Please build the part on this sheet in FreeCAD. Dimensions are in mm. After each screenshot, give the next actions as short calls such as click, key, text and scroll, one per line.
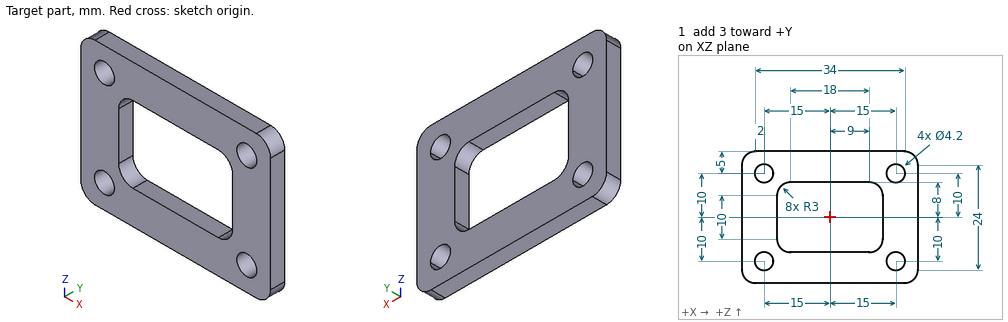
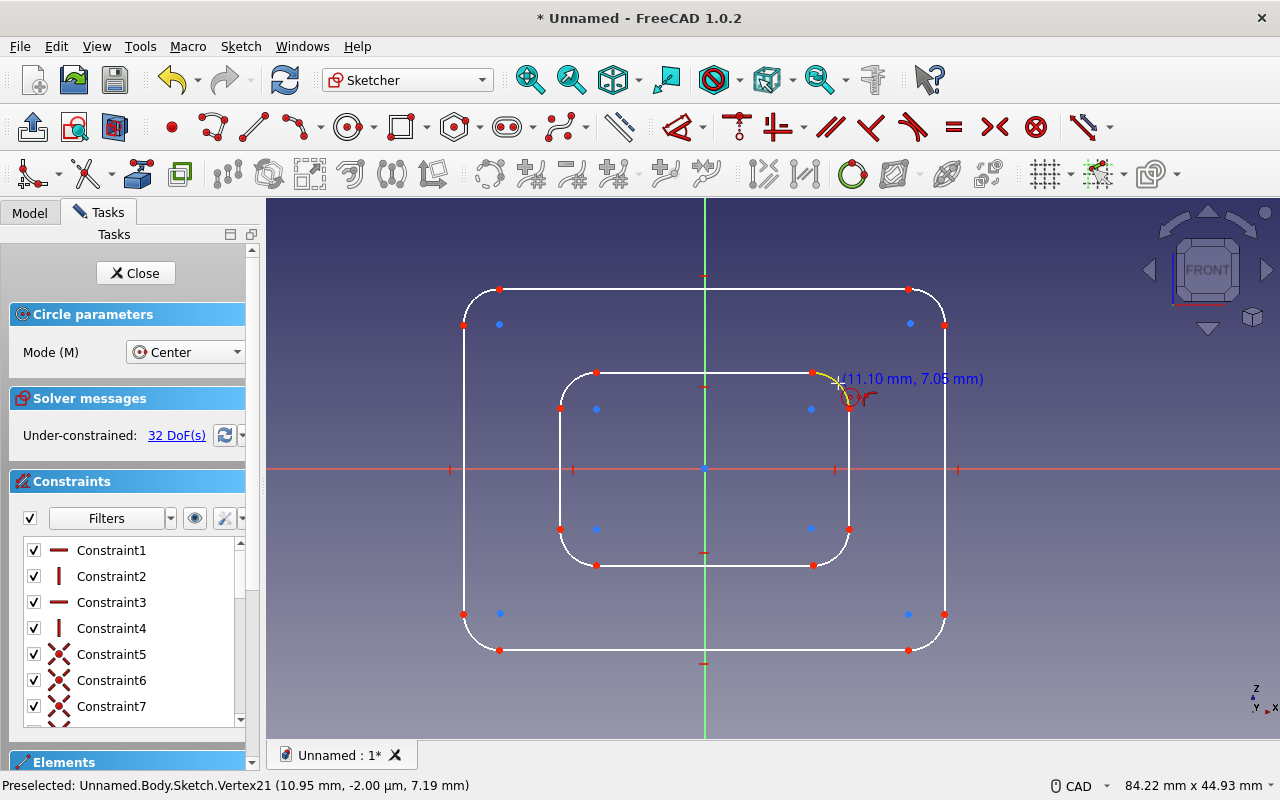
click(524, 348)
move(542, 330)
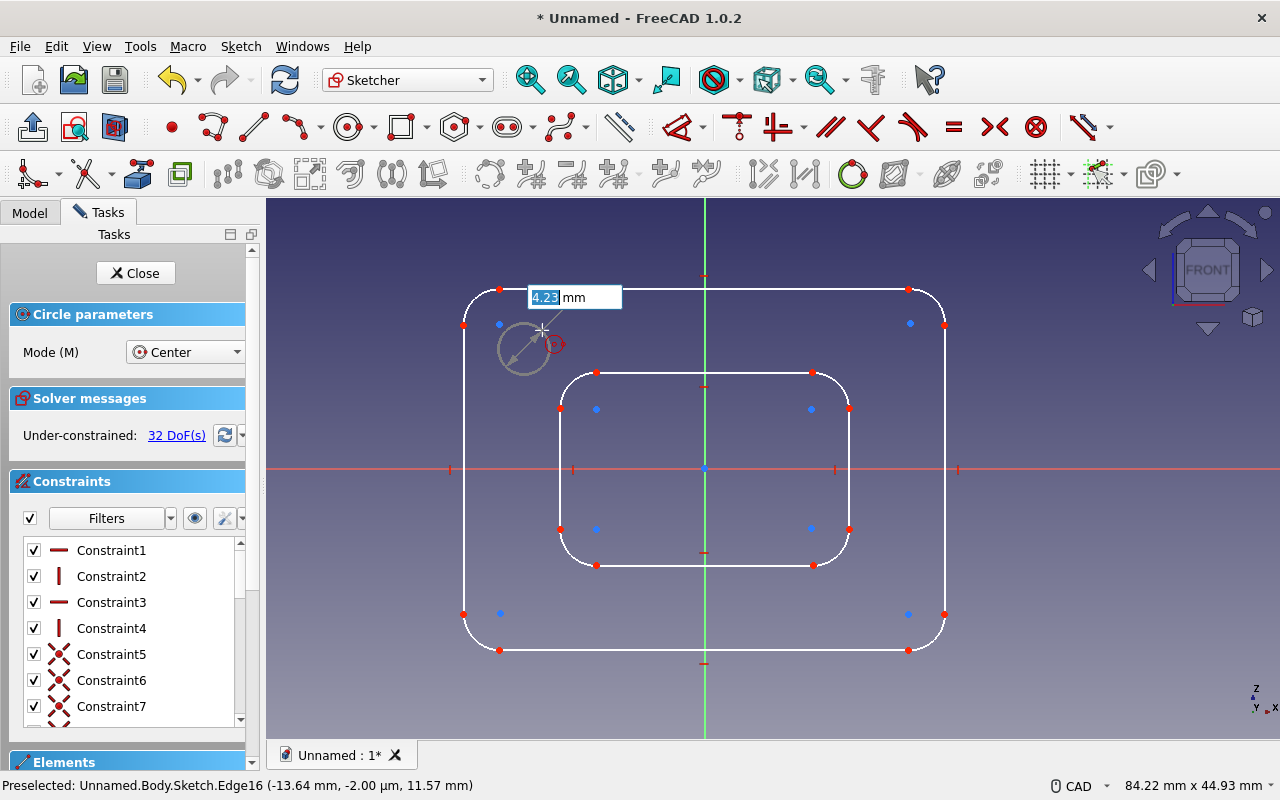
text(4.2)
key(Return)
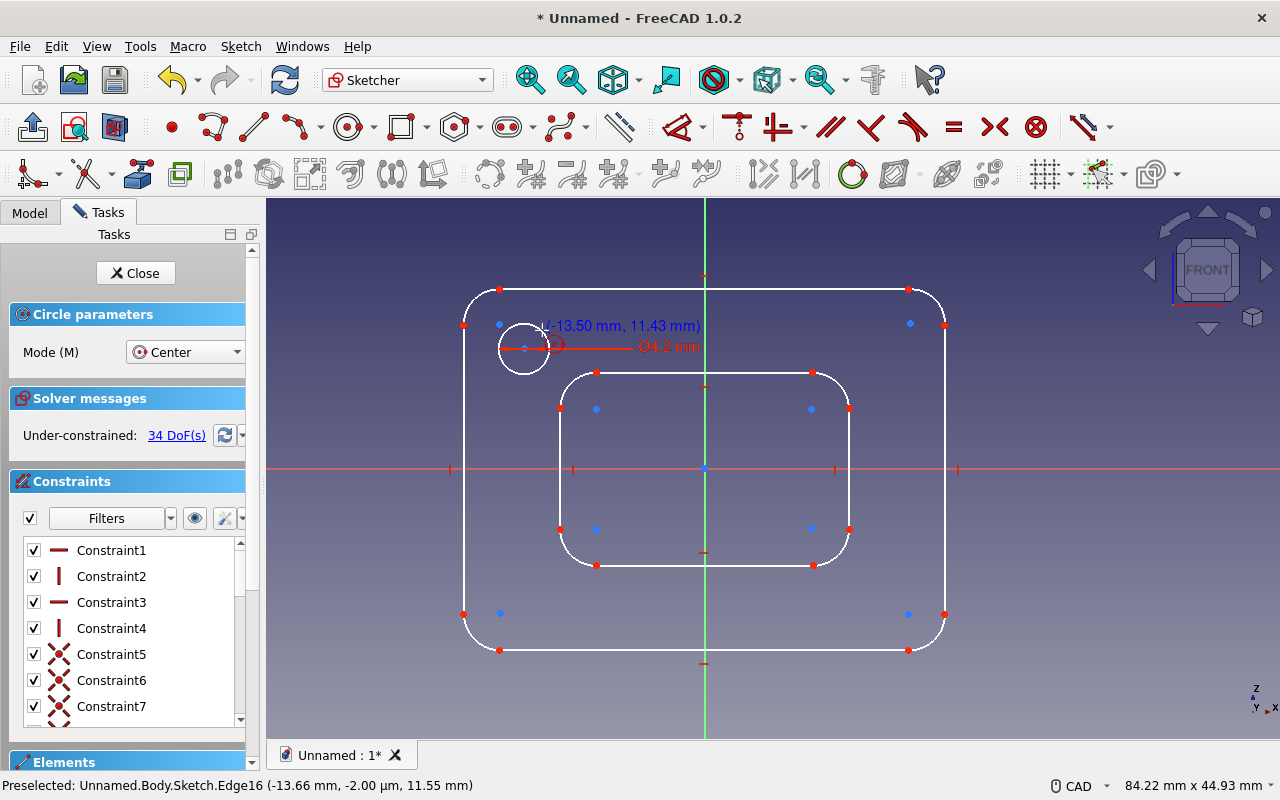
click(885, 348)
move(867, 330)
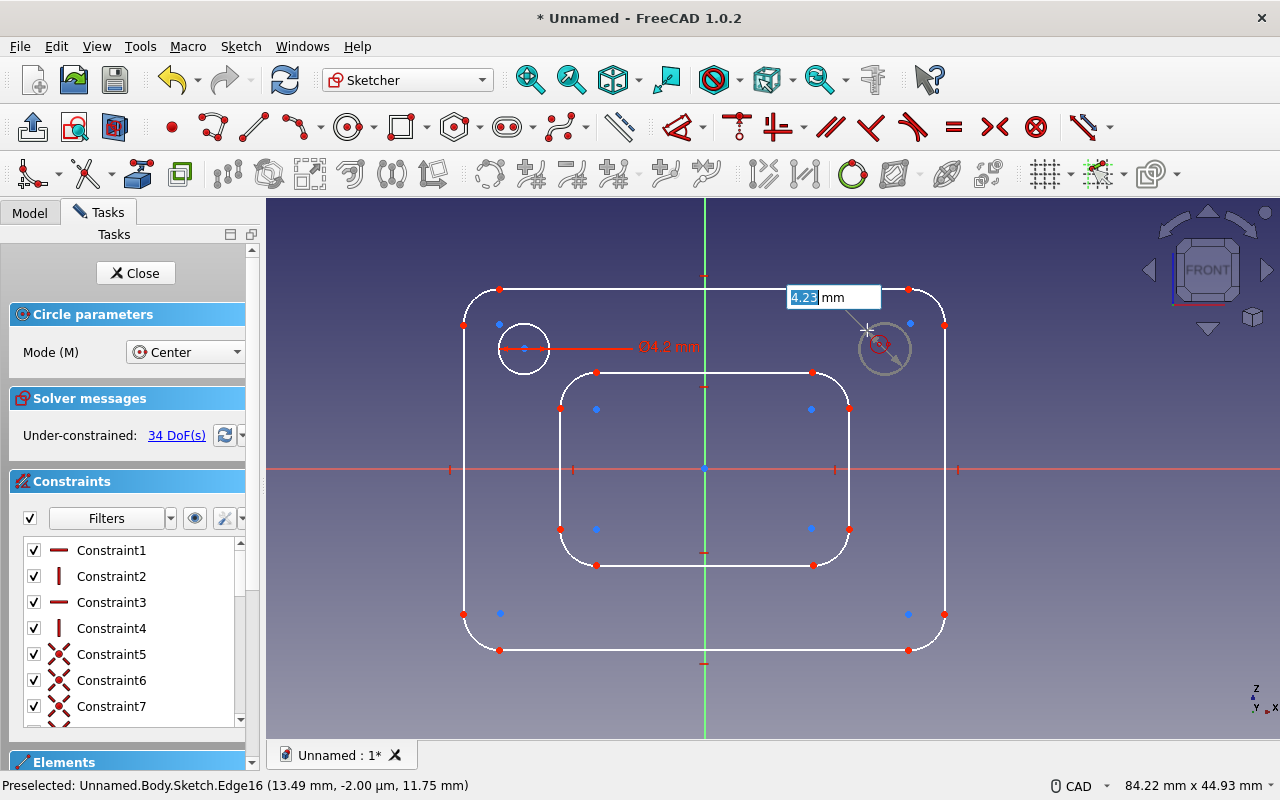
text(4.2)
key(Return)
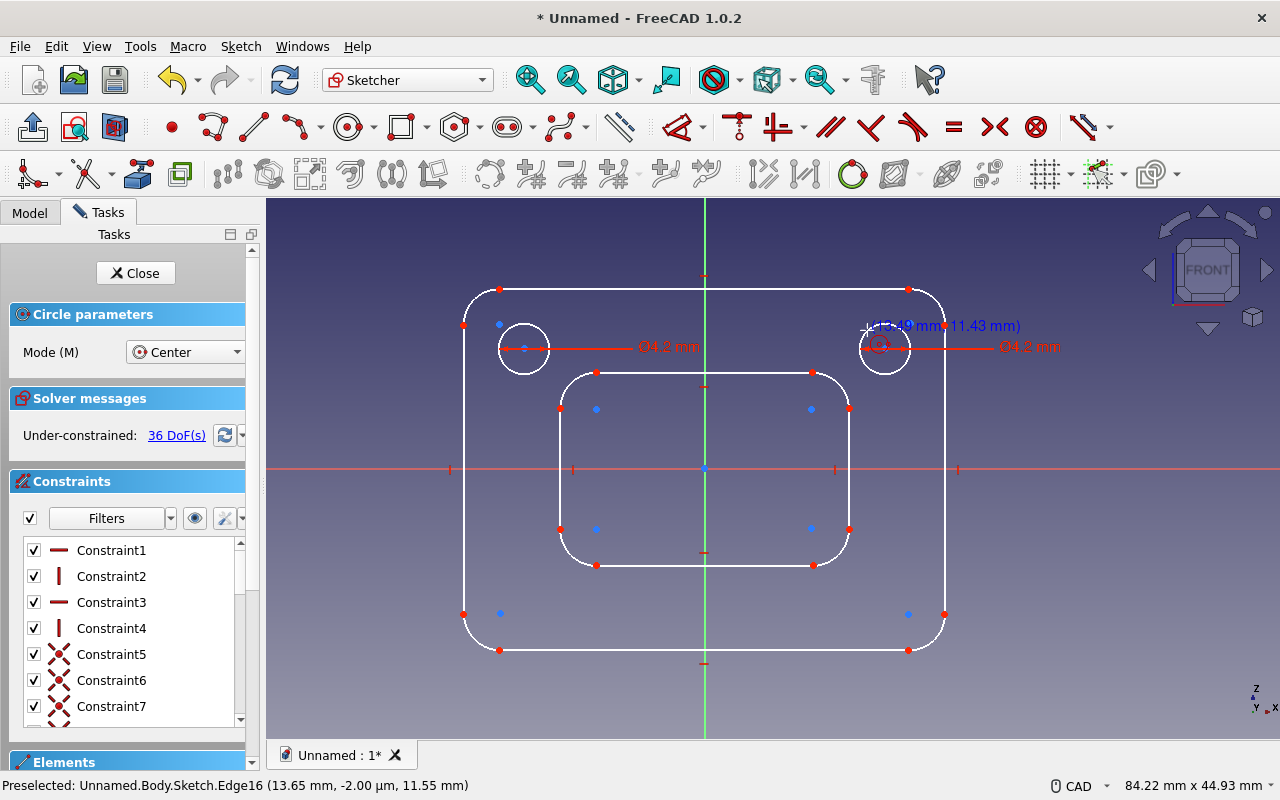
click(524, 589)
move(542, 571)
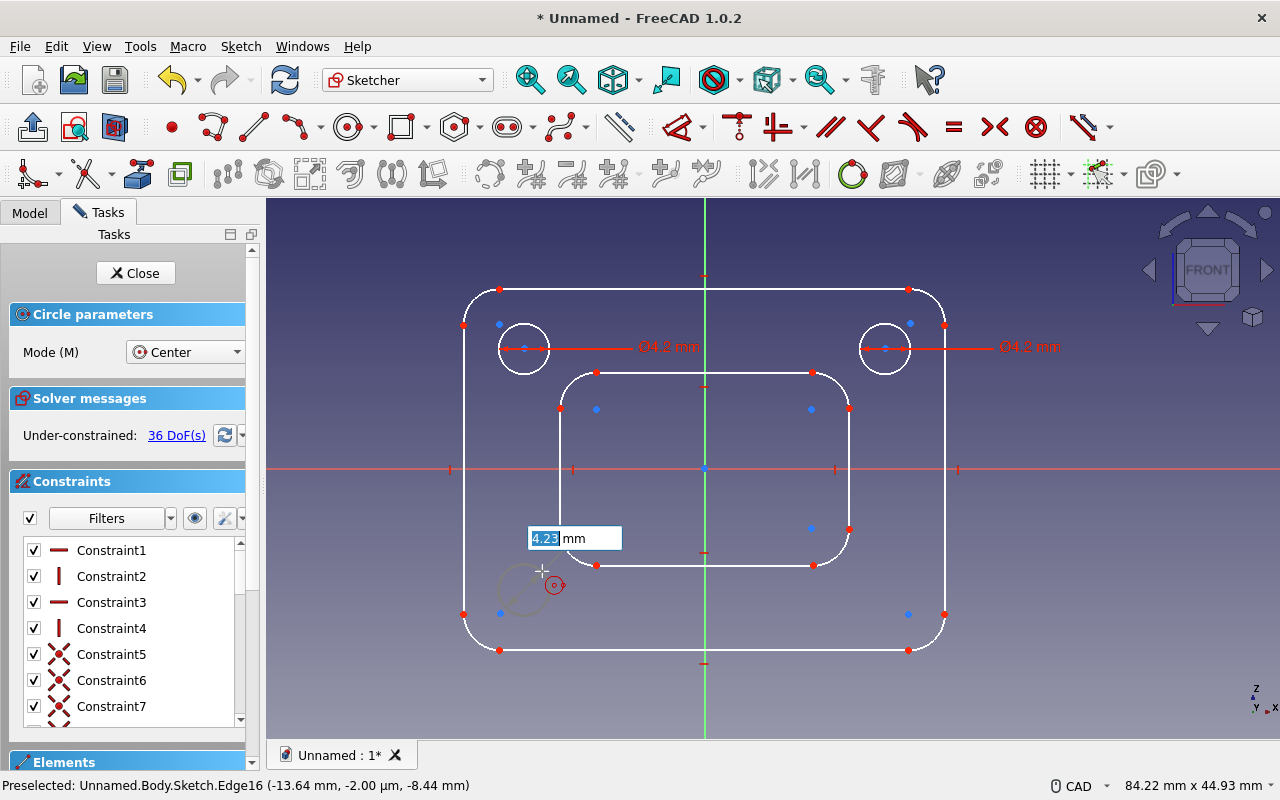
text(4.2)
key(Return)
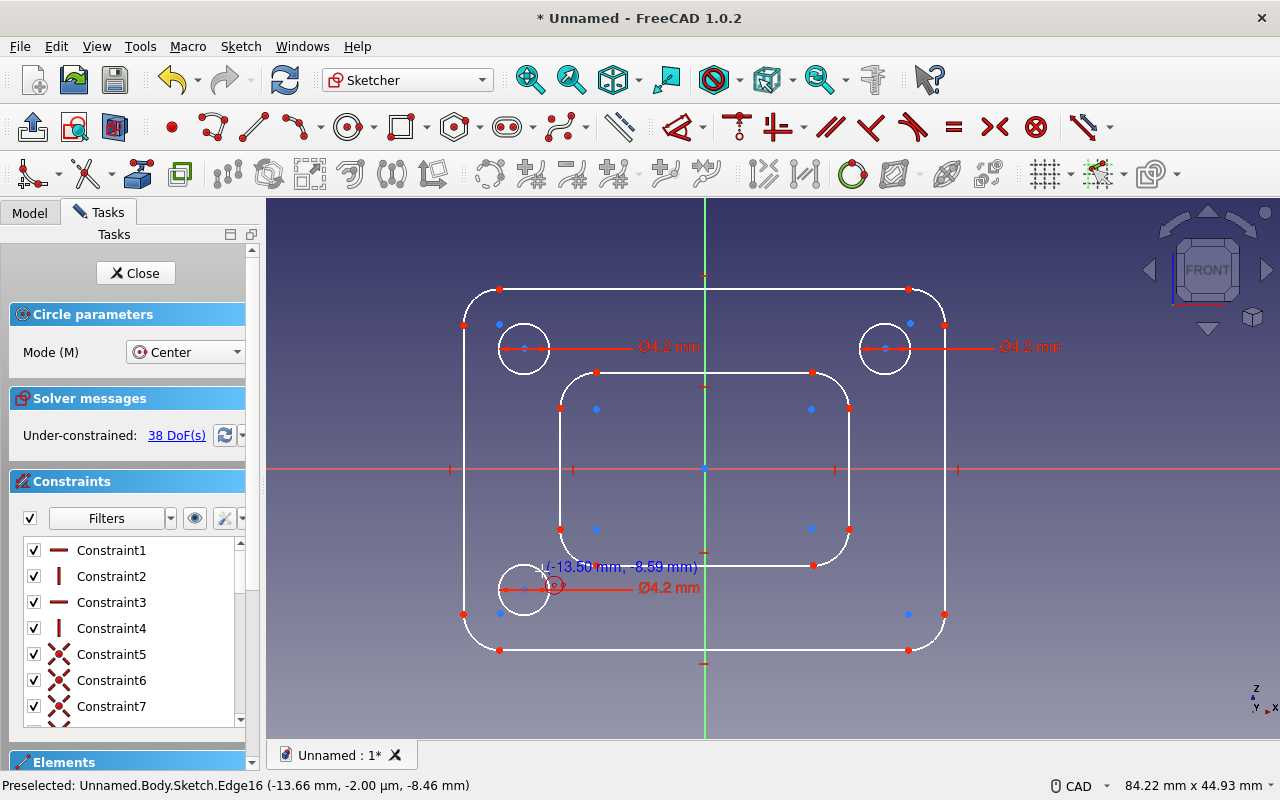
click(885, 589)
move(903, 571)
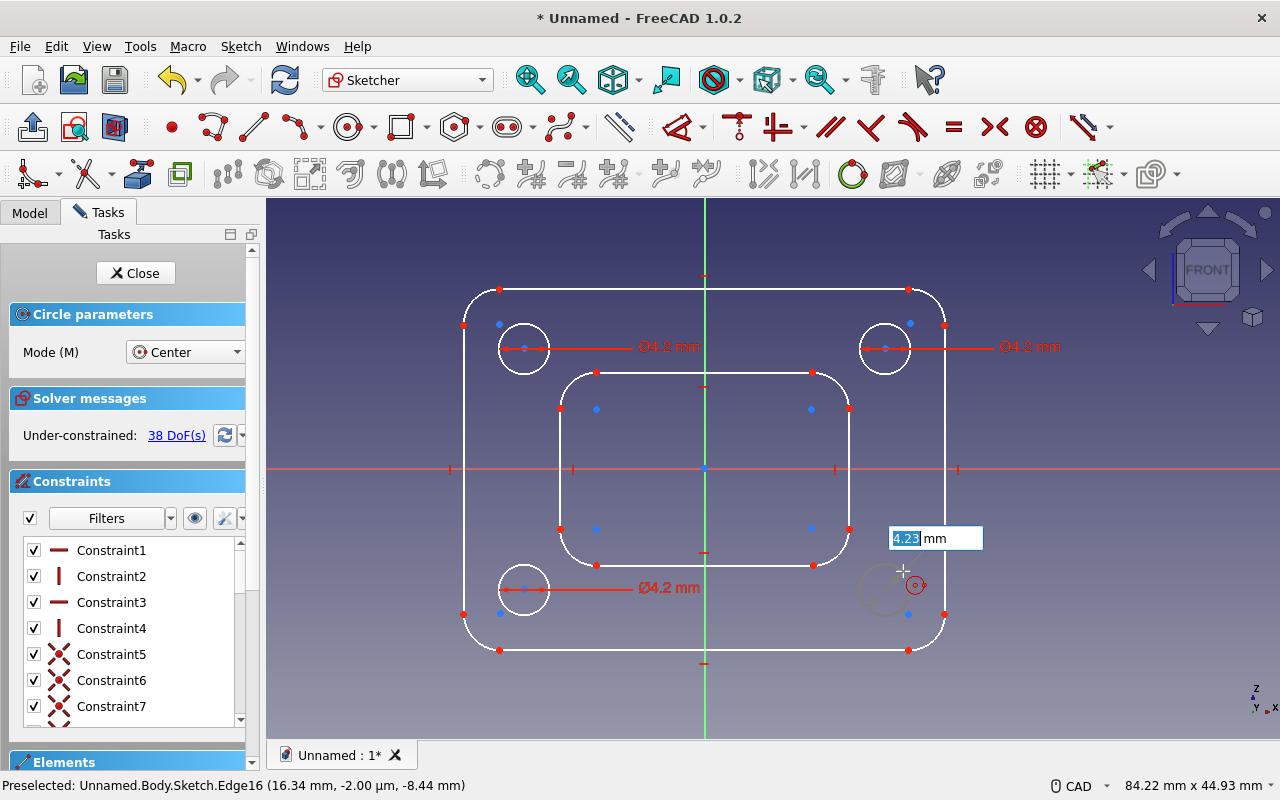
text(4.2)
key(Return)
key(Escape)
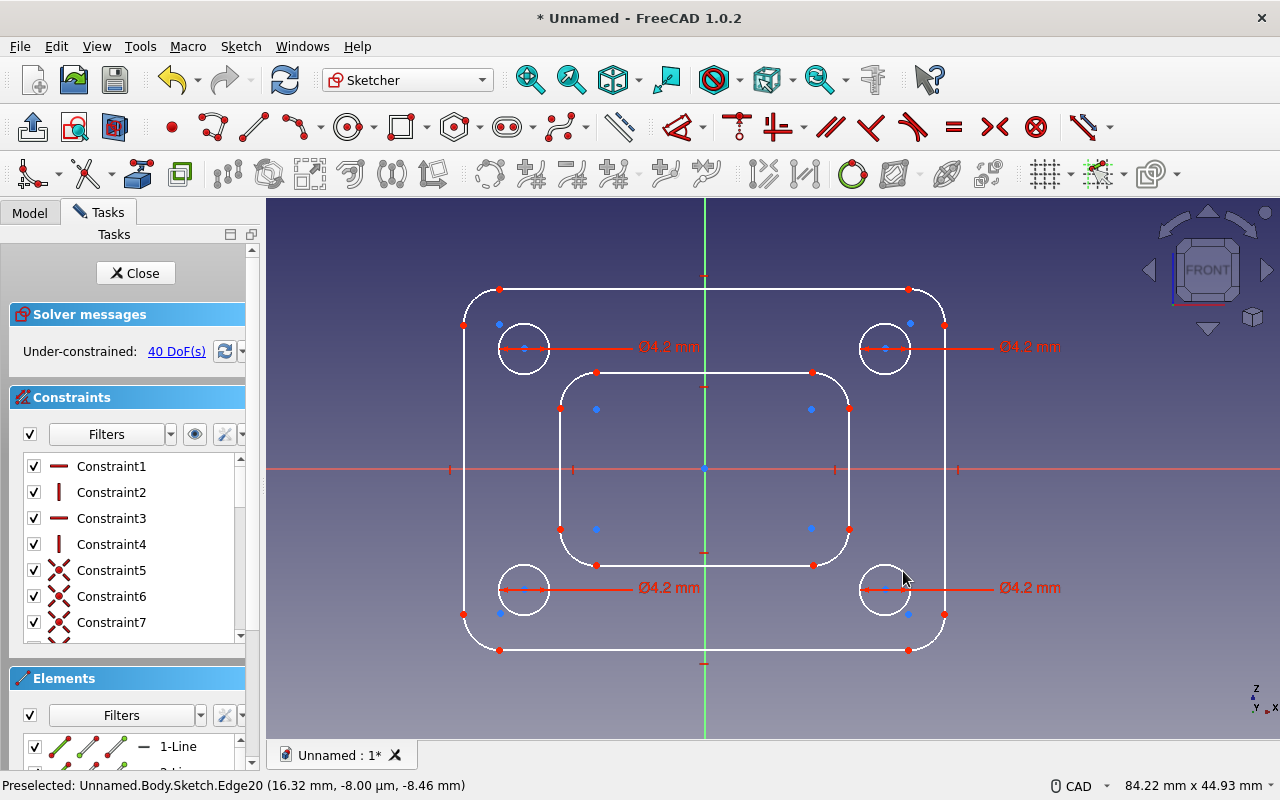
click(623, 289)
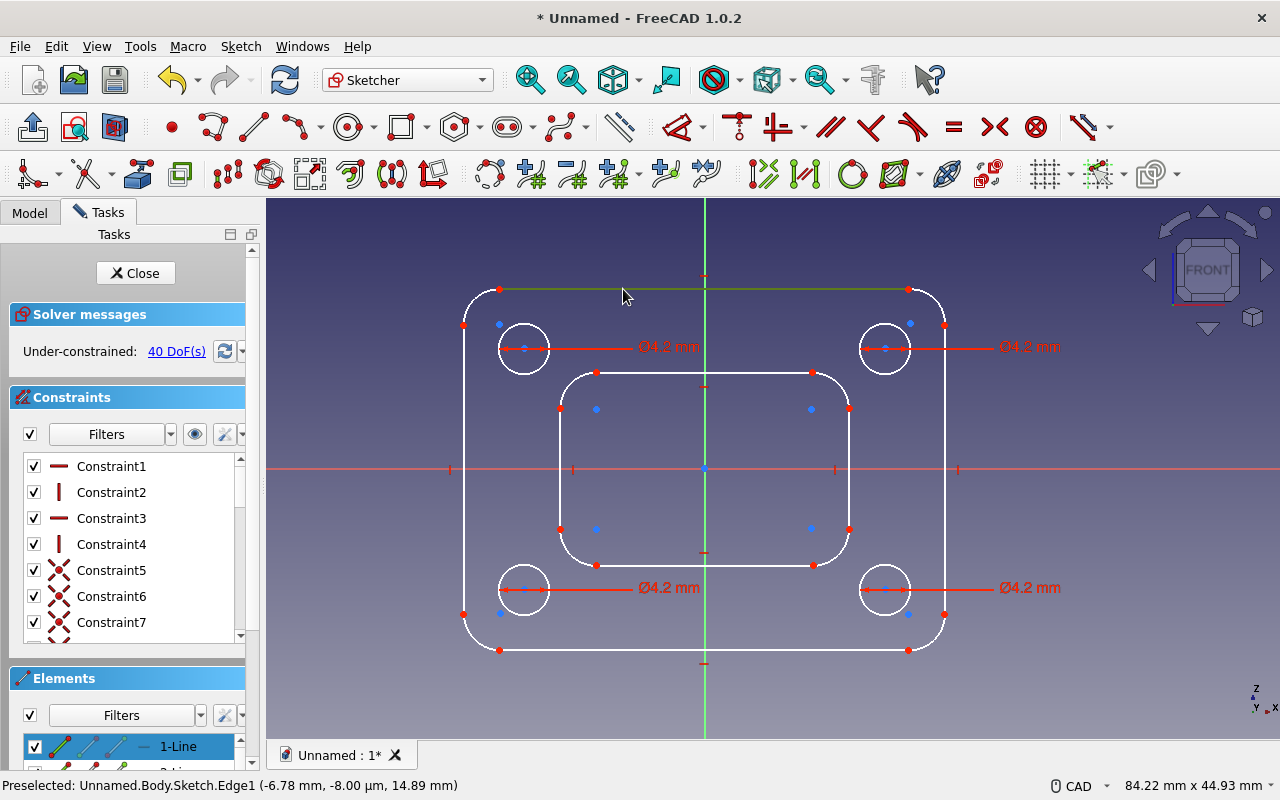
click(942, 309)